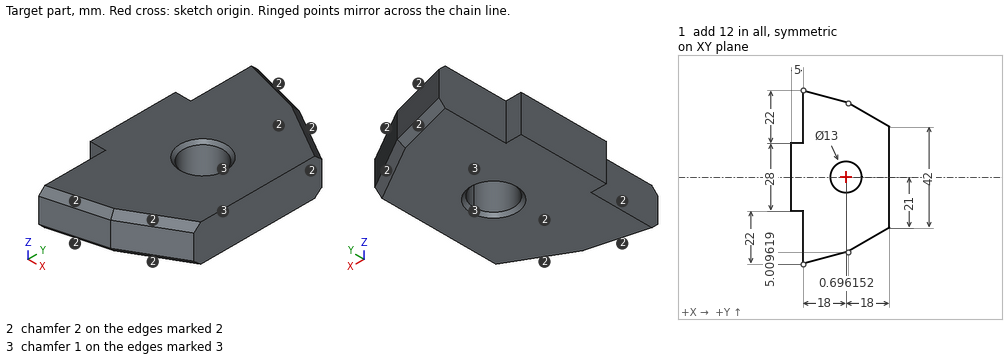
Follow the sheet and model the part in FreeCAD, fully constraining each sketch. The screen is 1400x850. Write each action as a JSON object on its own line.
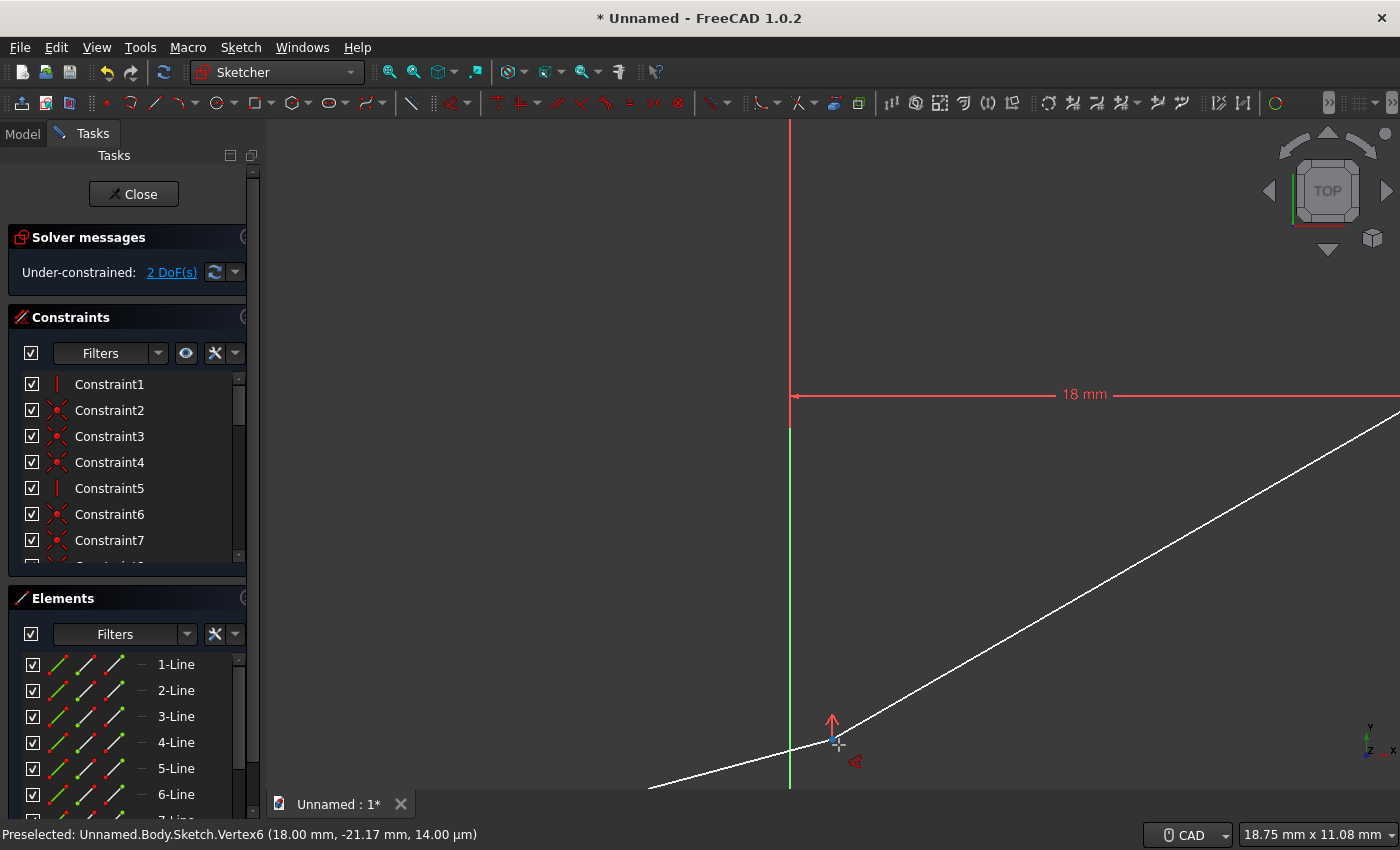
{"action": "left_click", "coordinate": [832, 739]}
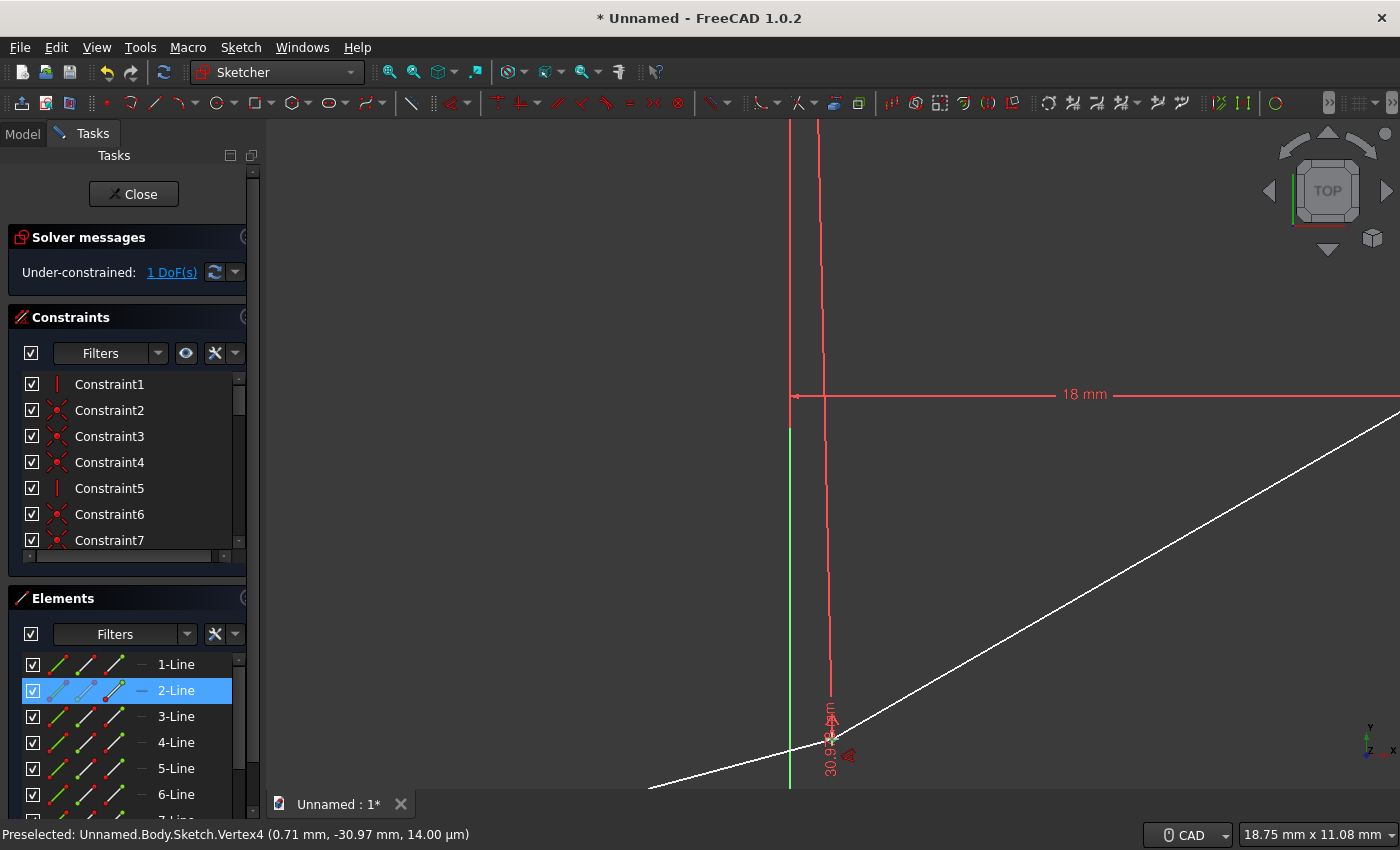
{"action": "key", "text": "Escape"}
{"action": "key", "text": "Escape"}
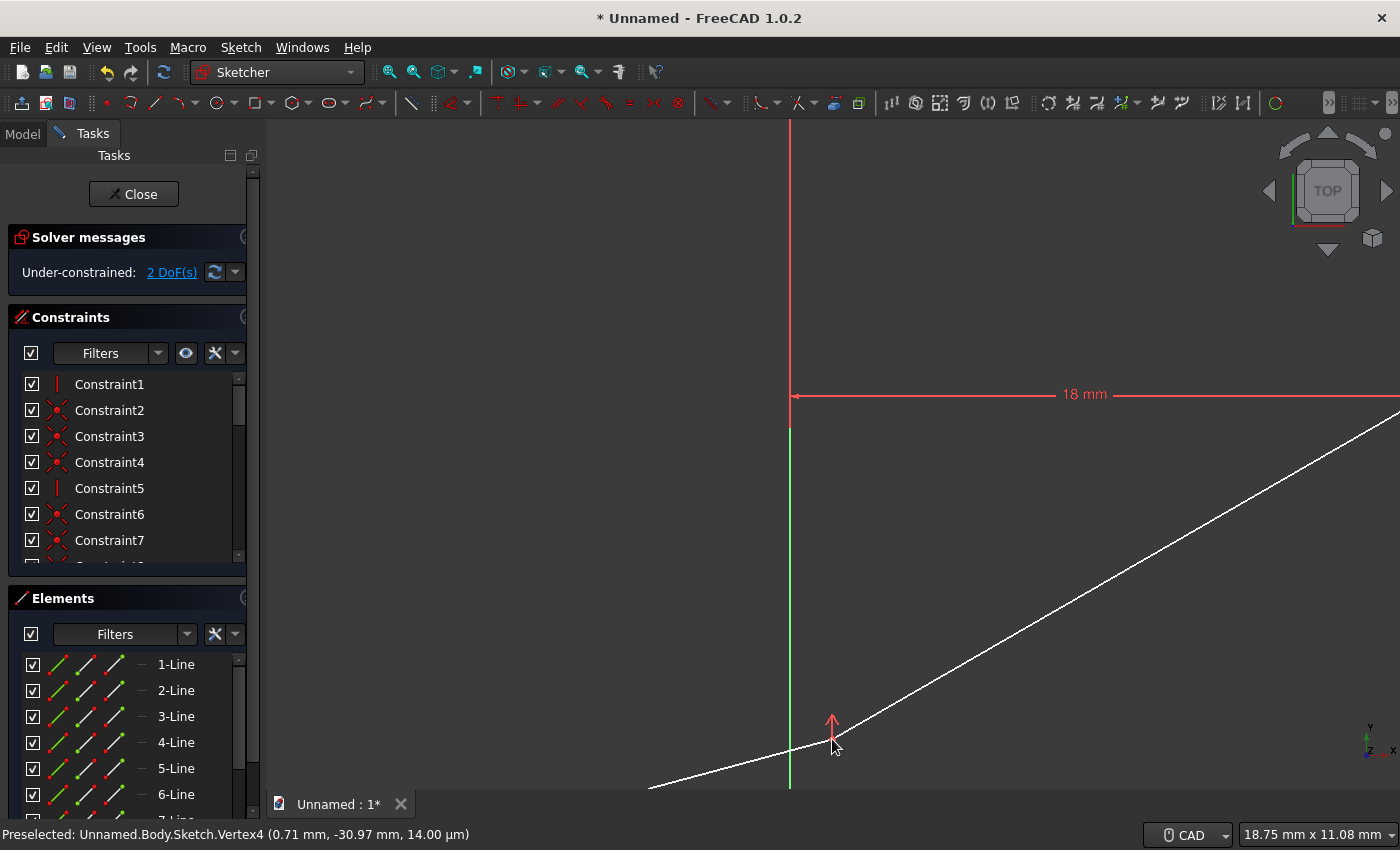
{"action": "left_click", "coordinate": [832, 739]}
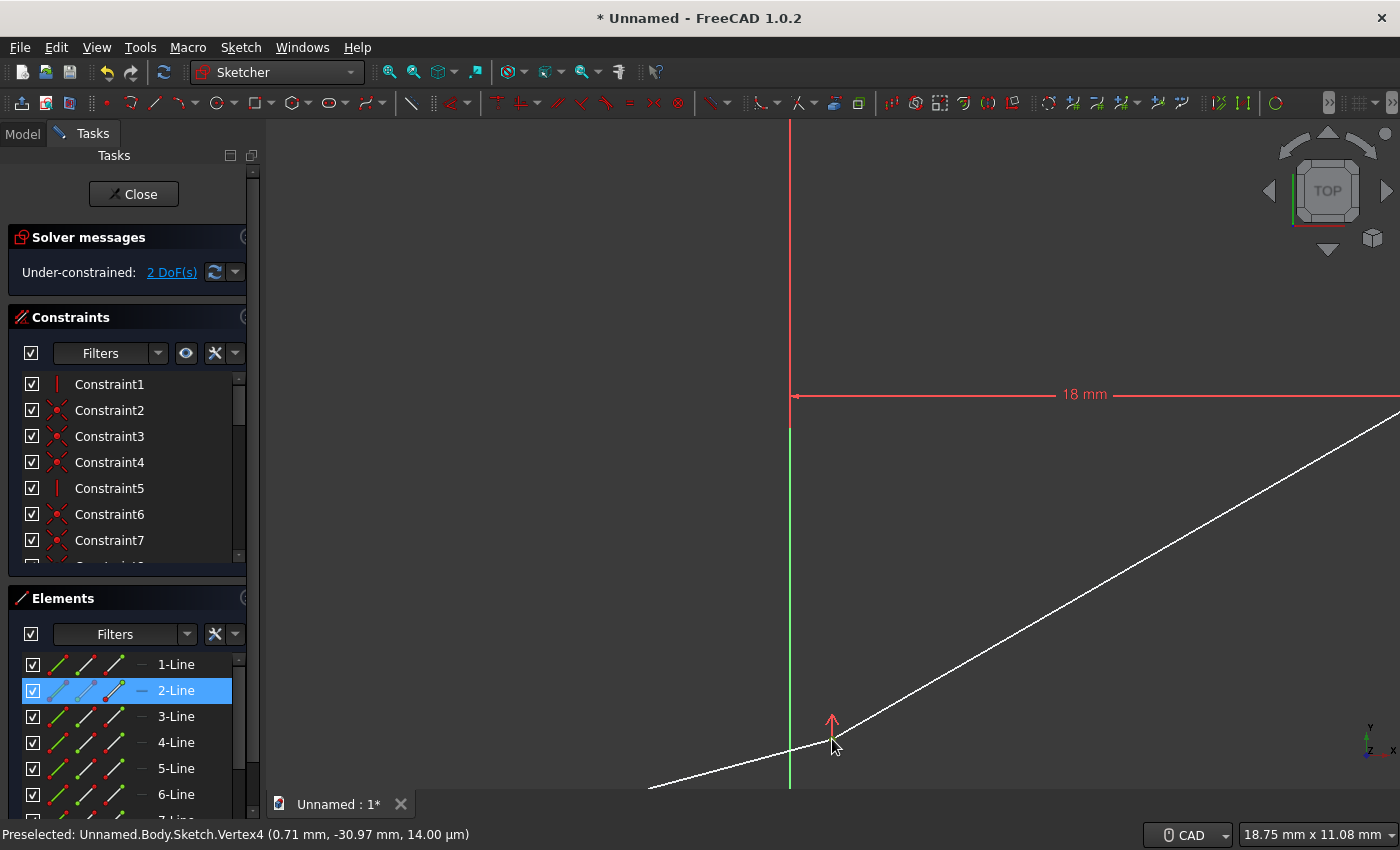
{"action": "left_click", "coordinate": [470, 104]}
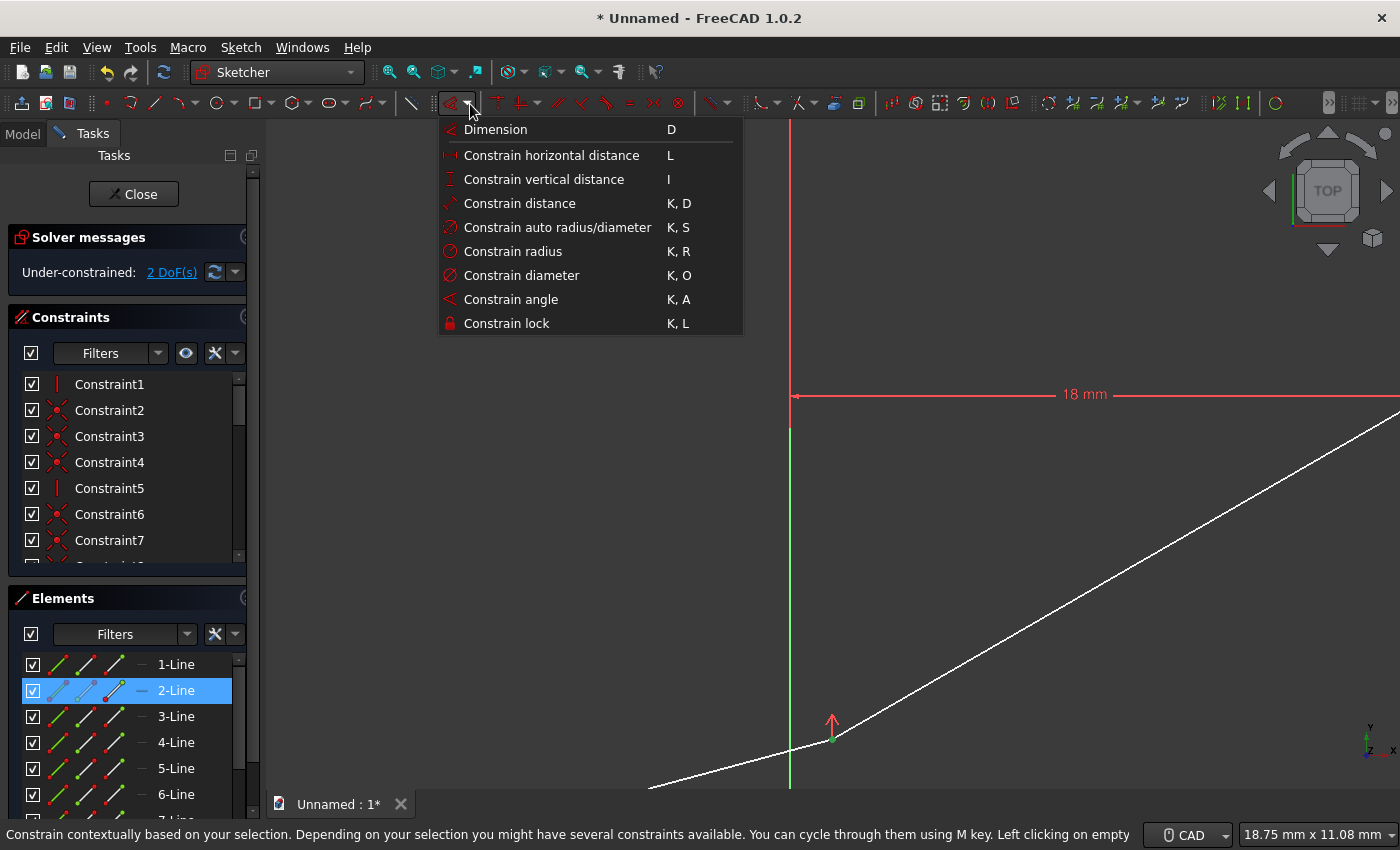
{"action": "left_click", "coordinate": [591, 155]}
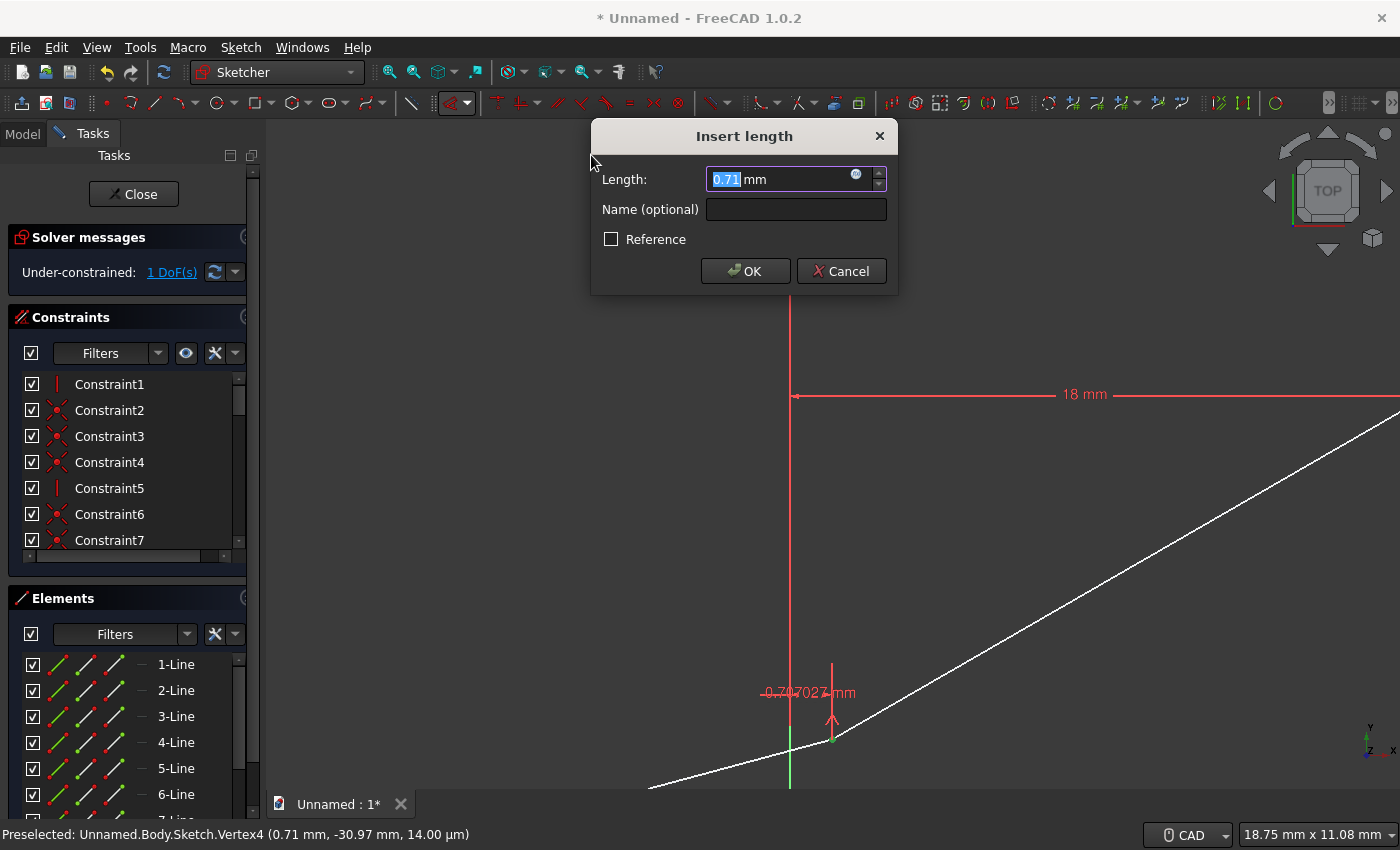
{"action": "type", "text": "0.696152"}
{"action": "key", "text": "Return"}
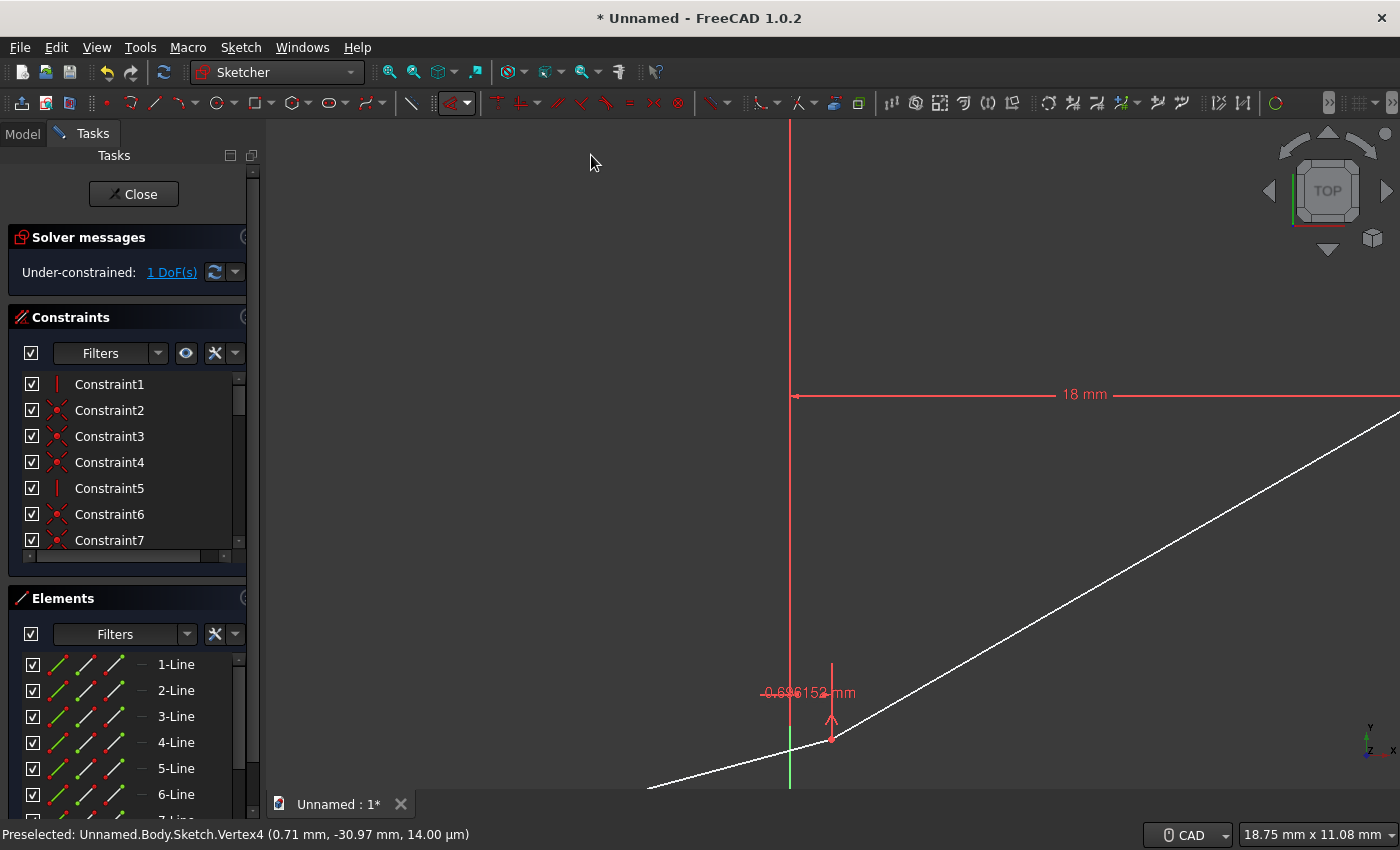
{"action": "scroll", "coordinate": [777, 612], "scroll_direction": "down", "scroll_amount": 12}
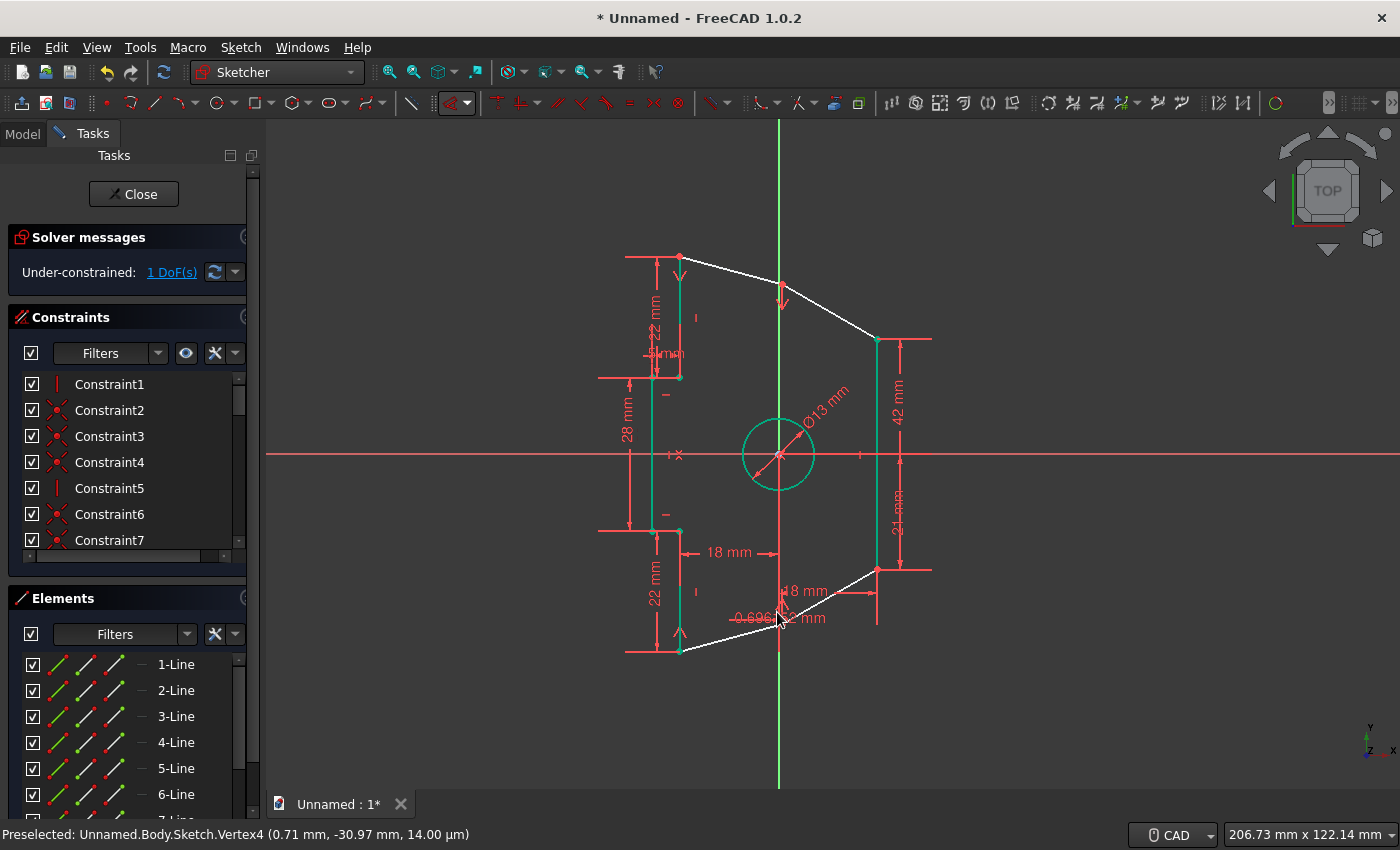
{"action": "scroll", "coordinate": [711, 644], "scroll_direction": "up", "scroll_amount": 2}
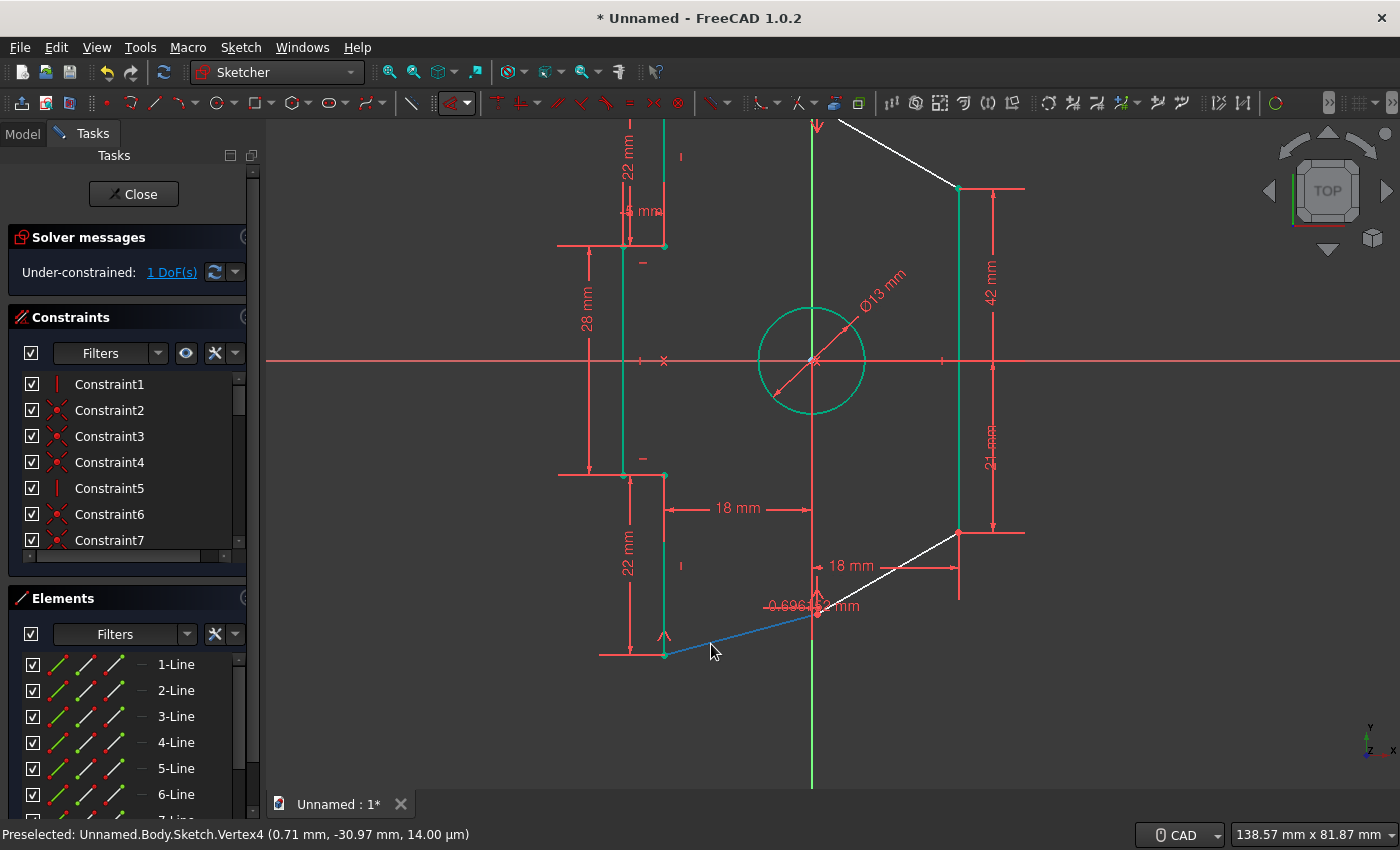
{"action": "left_click", "coordinate": [710, 643]}